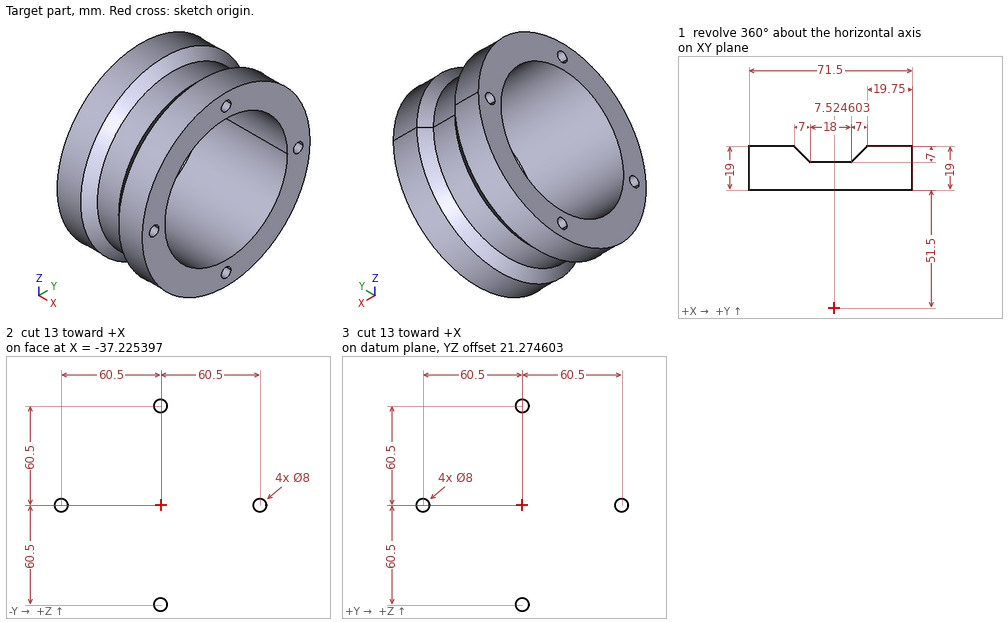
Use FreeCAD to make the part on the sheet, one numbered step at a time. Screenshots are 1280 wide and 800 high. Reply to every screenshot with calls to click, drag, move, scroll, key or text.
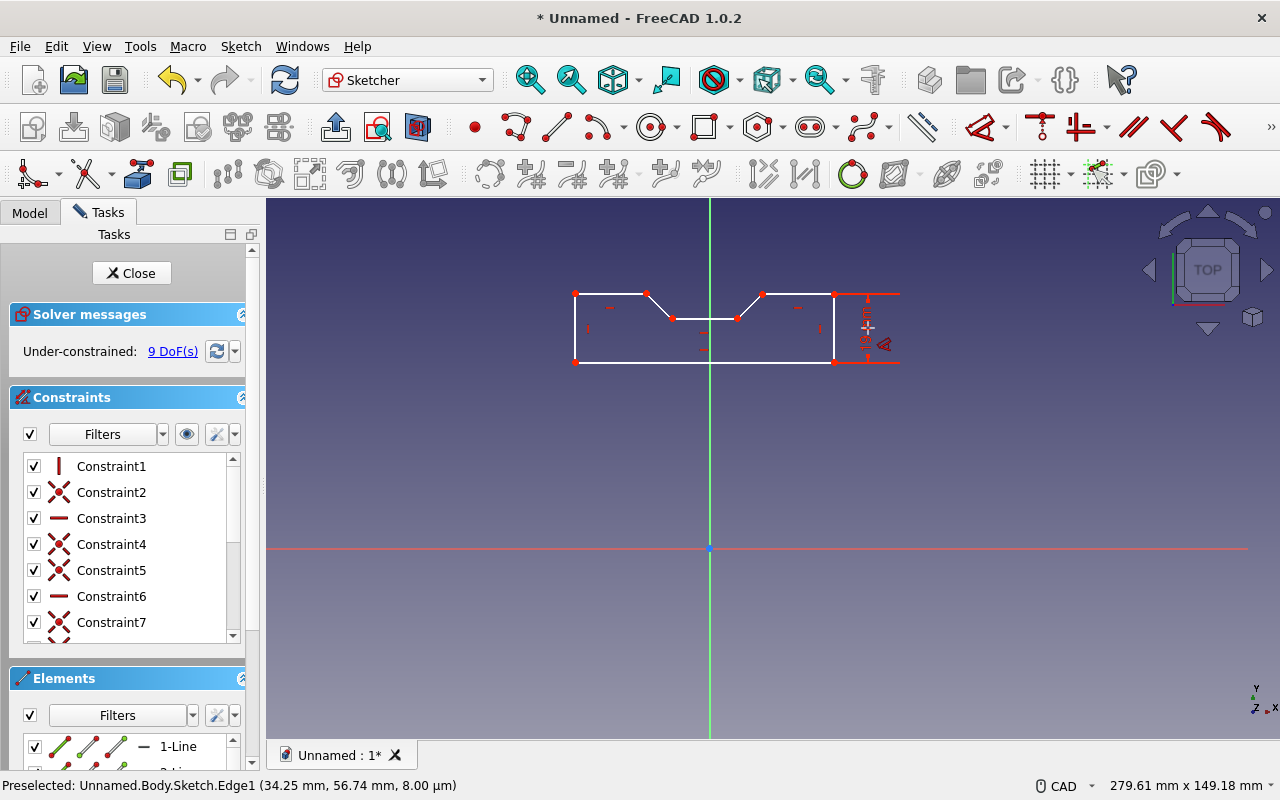
click(691, 319)
click(690, 285)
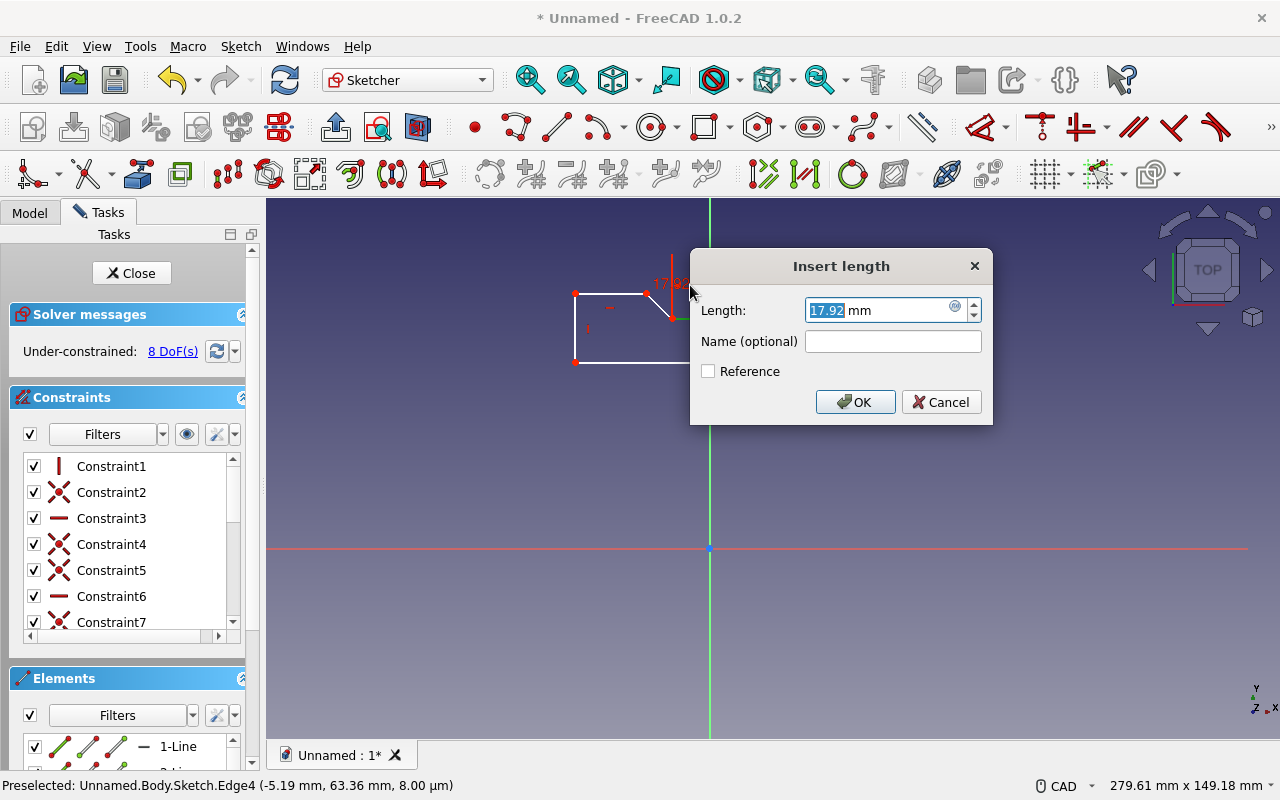
text(18)
key(Return)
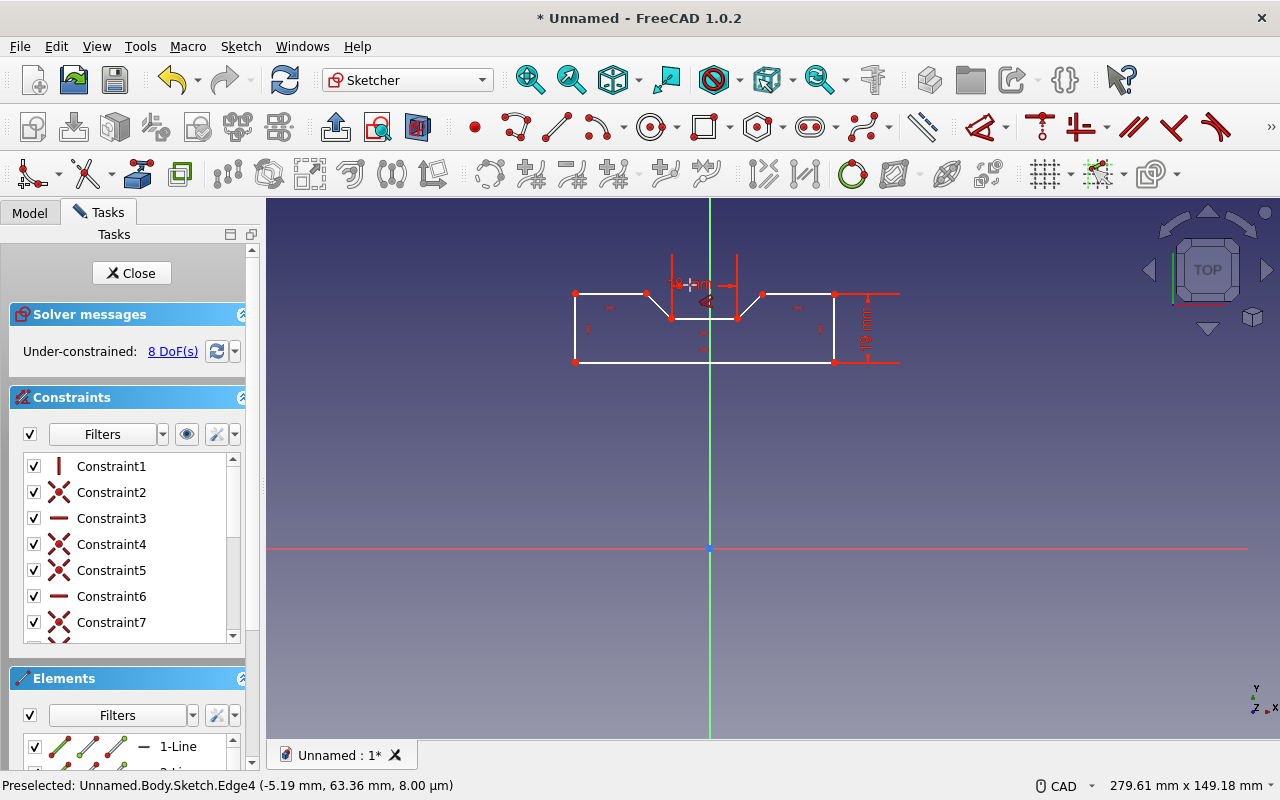
click(575, 315)
click(541, 328)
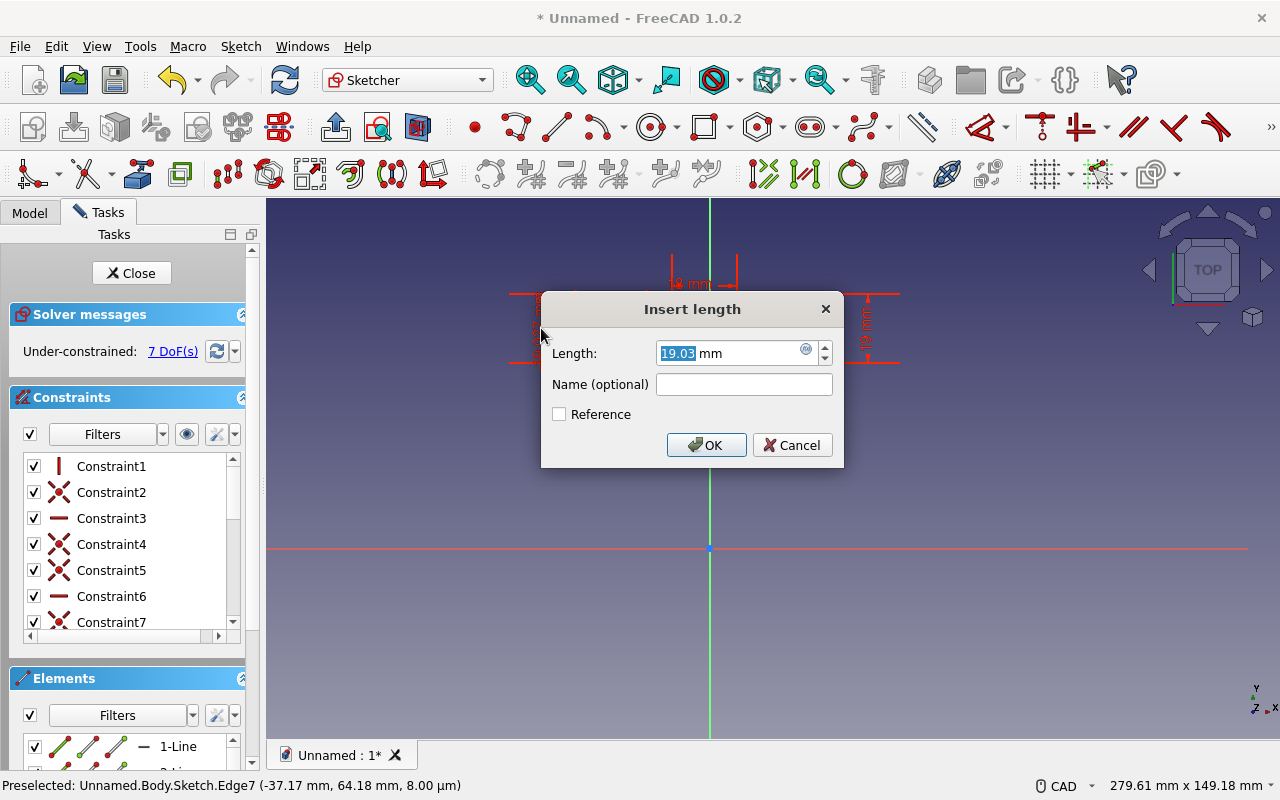
text(19)
key(Return)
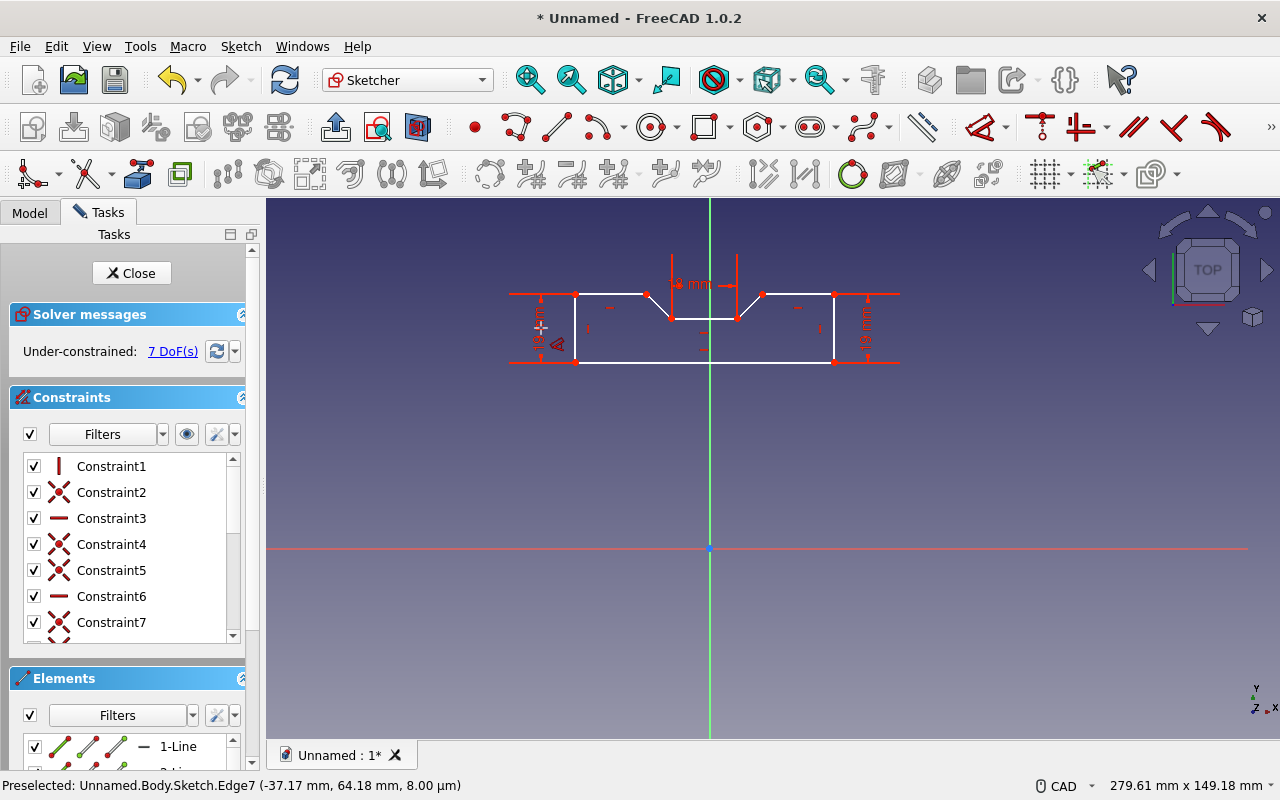
scroll(754, 302, up, 3)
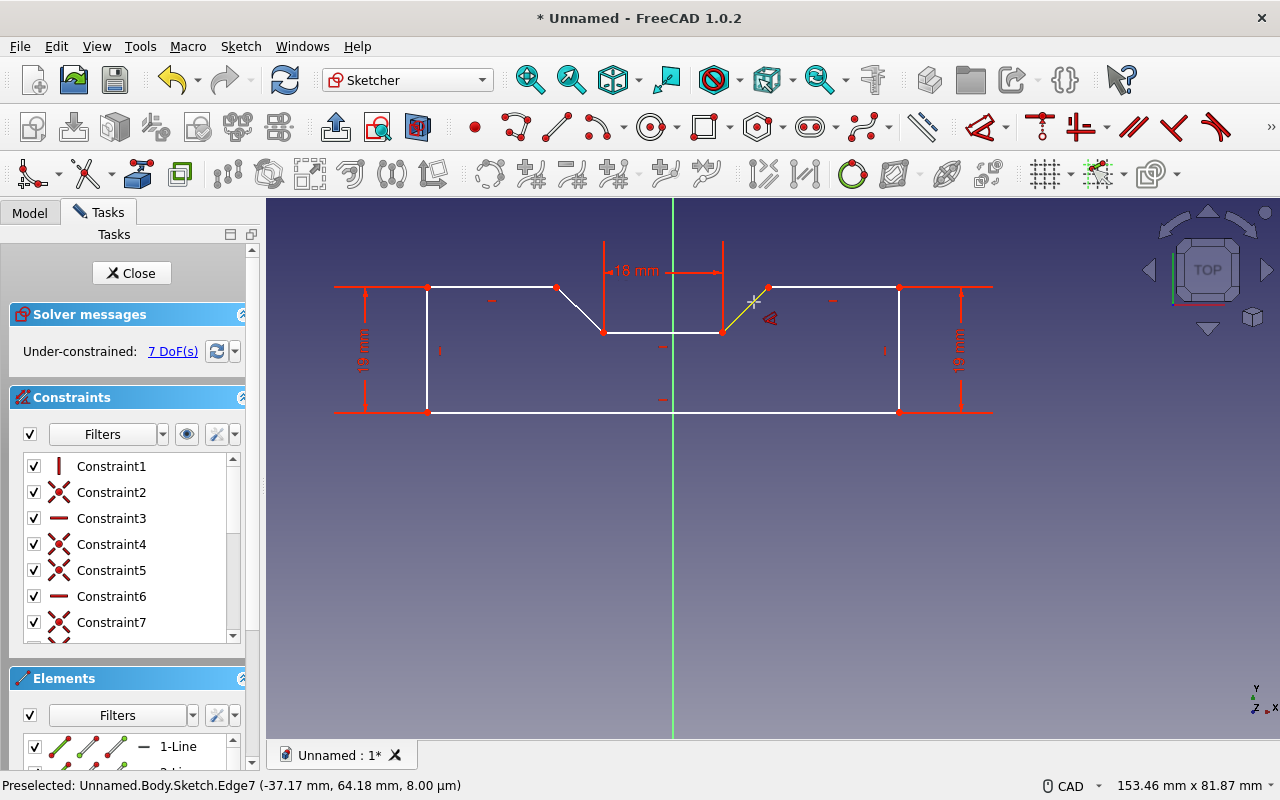
click(755, 301)
click(745, 253)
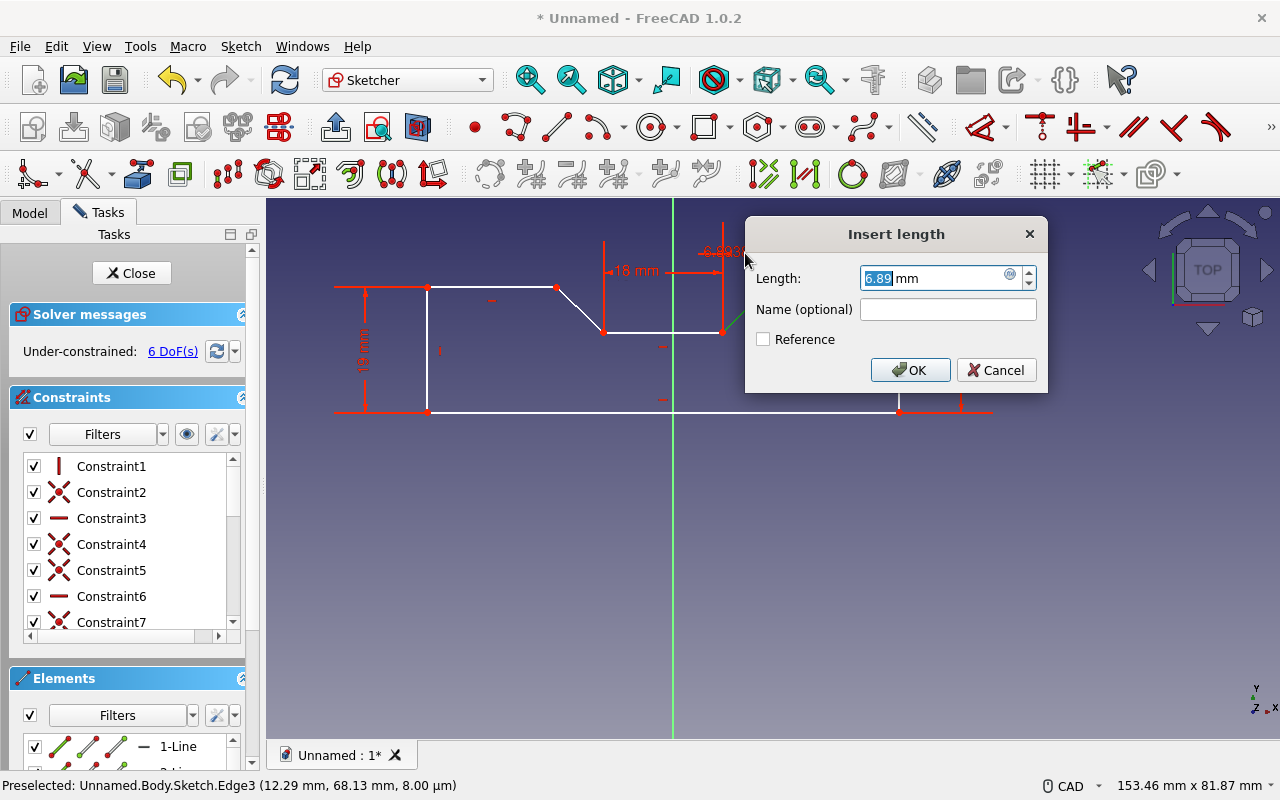
text(7)
key(Return)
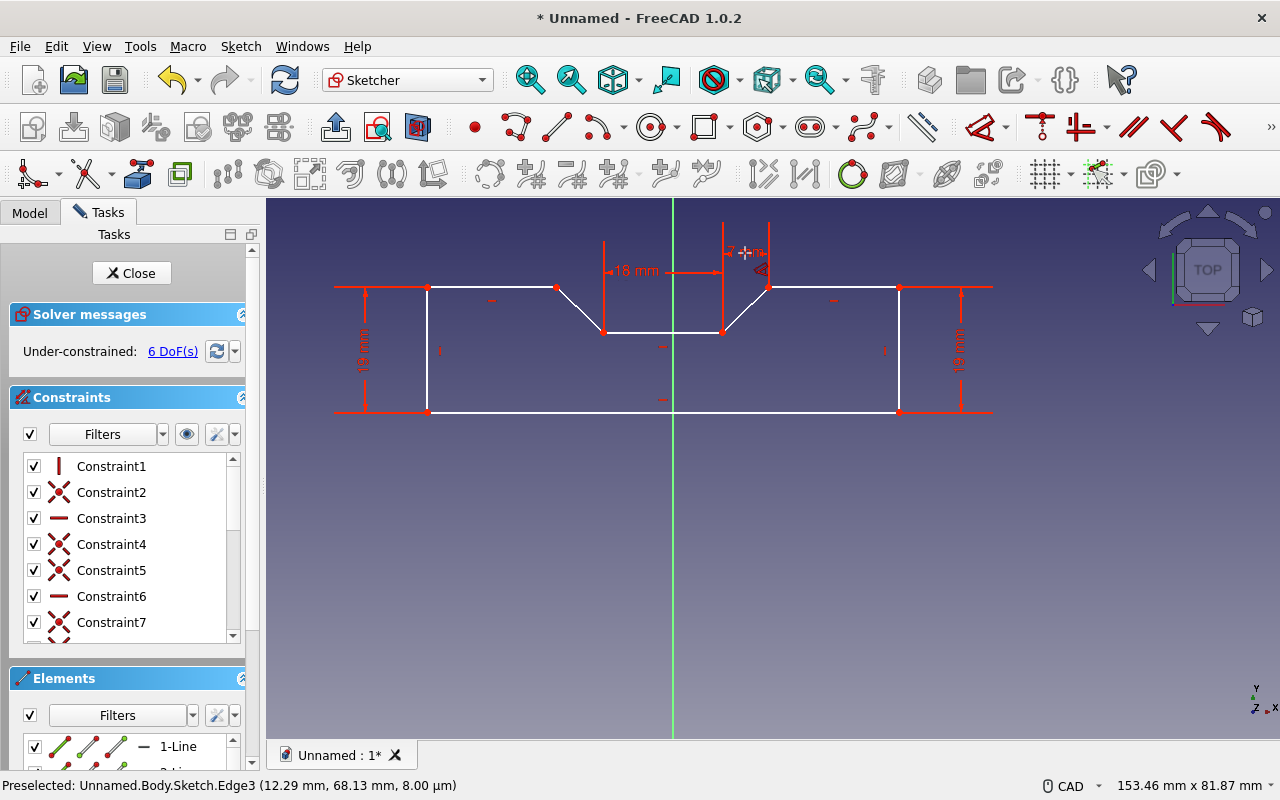
click(755, 301)
click(803, 310)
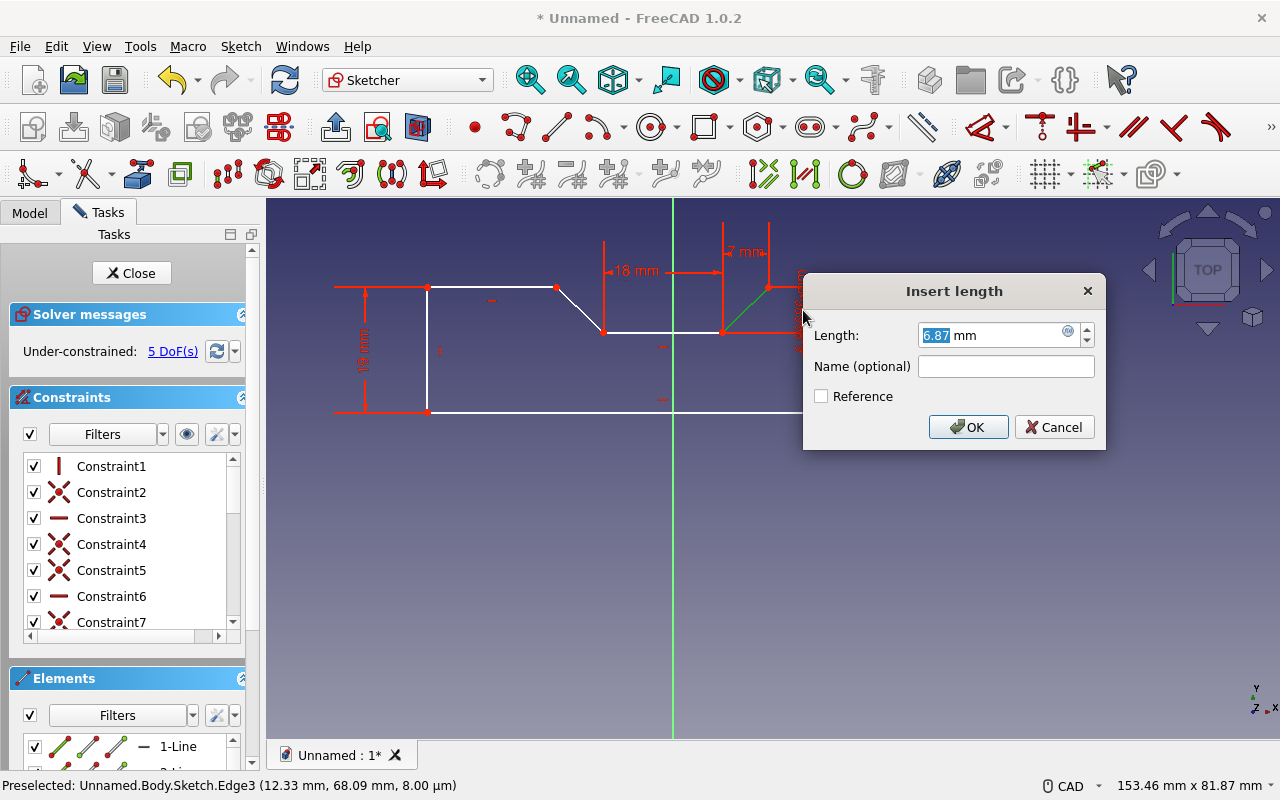
text(7)
key(Return)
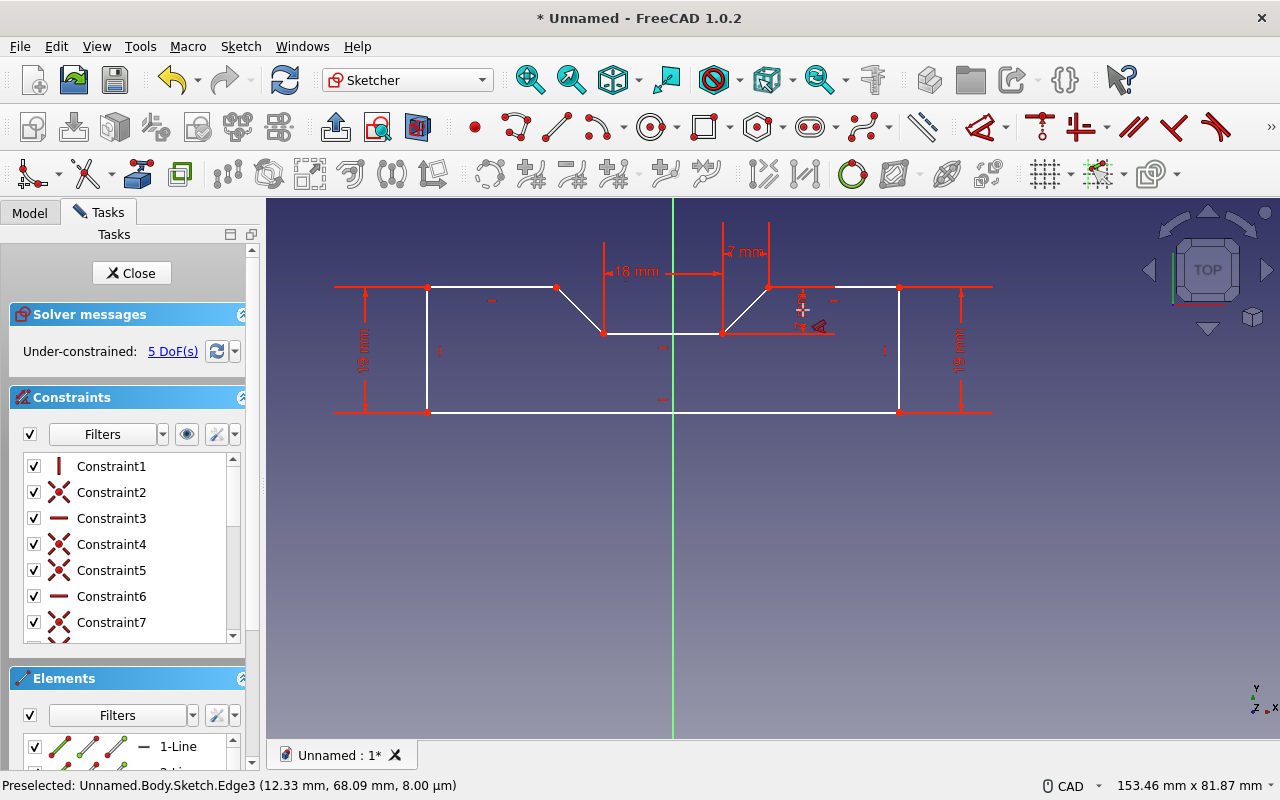
click(590, 320)
click(564, 253)